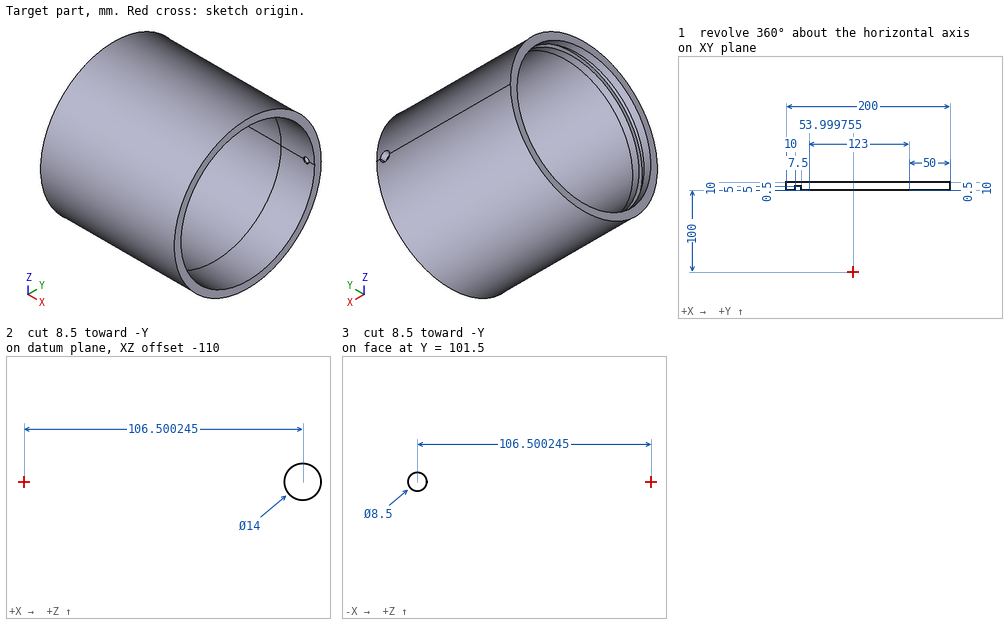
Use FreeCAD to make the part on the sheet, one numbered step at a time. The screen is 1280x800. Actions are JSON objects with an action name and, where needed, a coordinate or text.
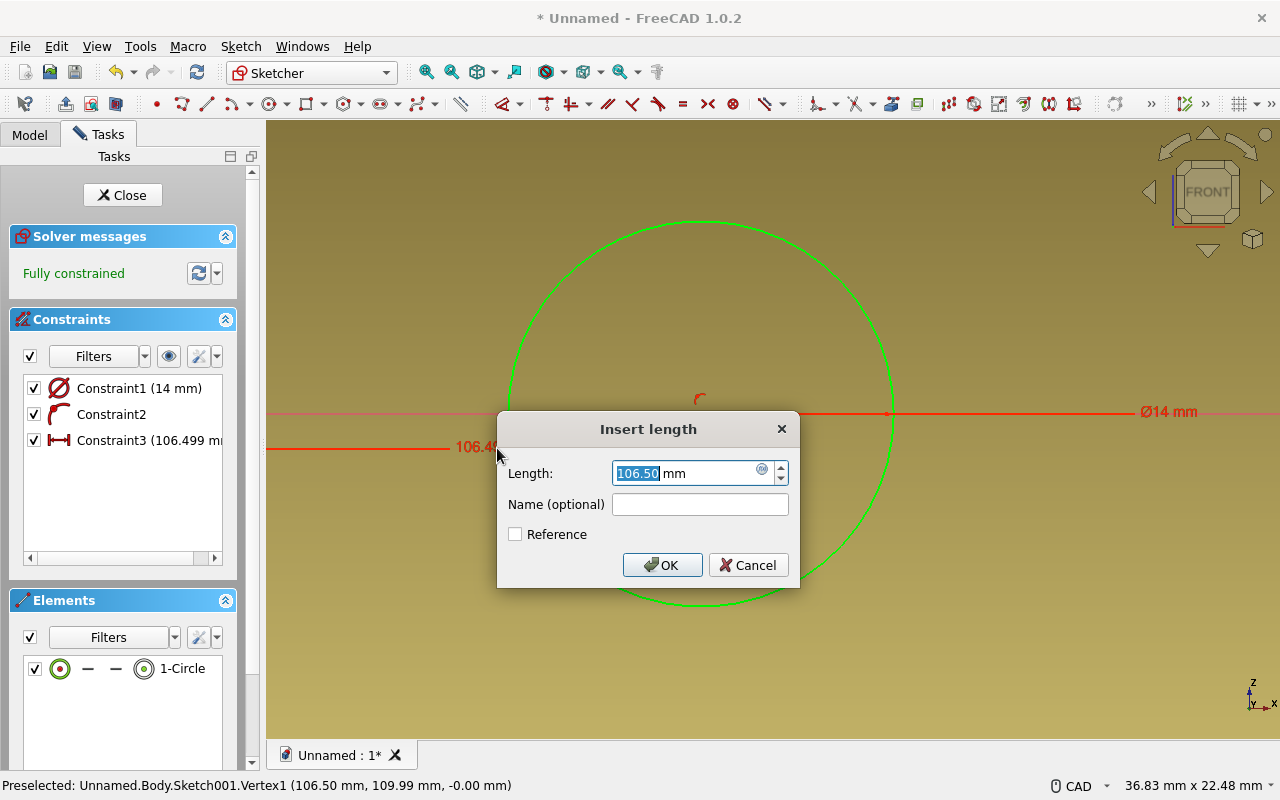
{"action": "type", "text": "106.500245"}
{"action": "key", "text": "Return"}
{"action": "key", "text": "Escape"}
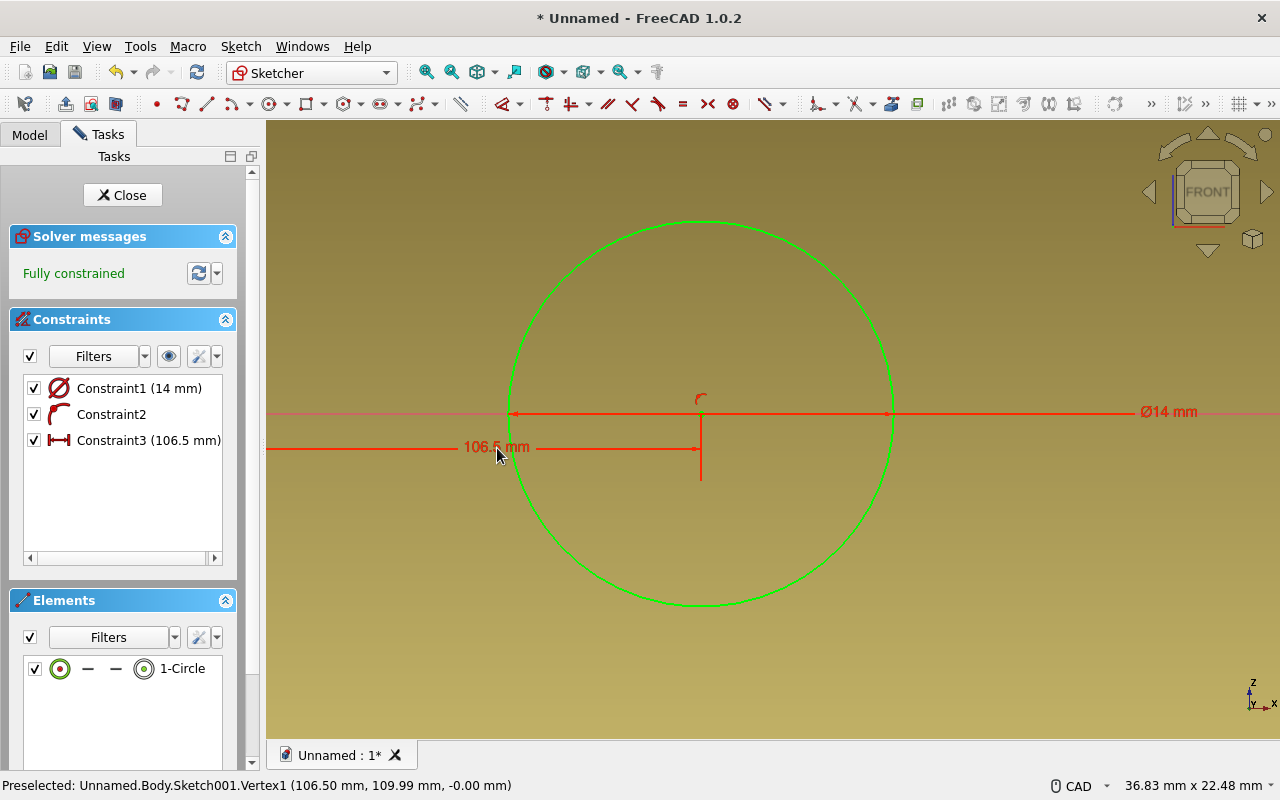
{"action": "left_click", "coordinate": [123, 195]}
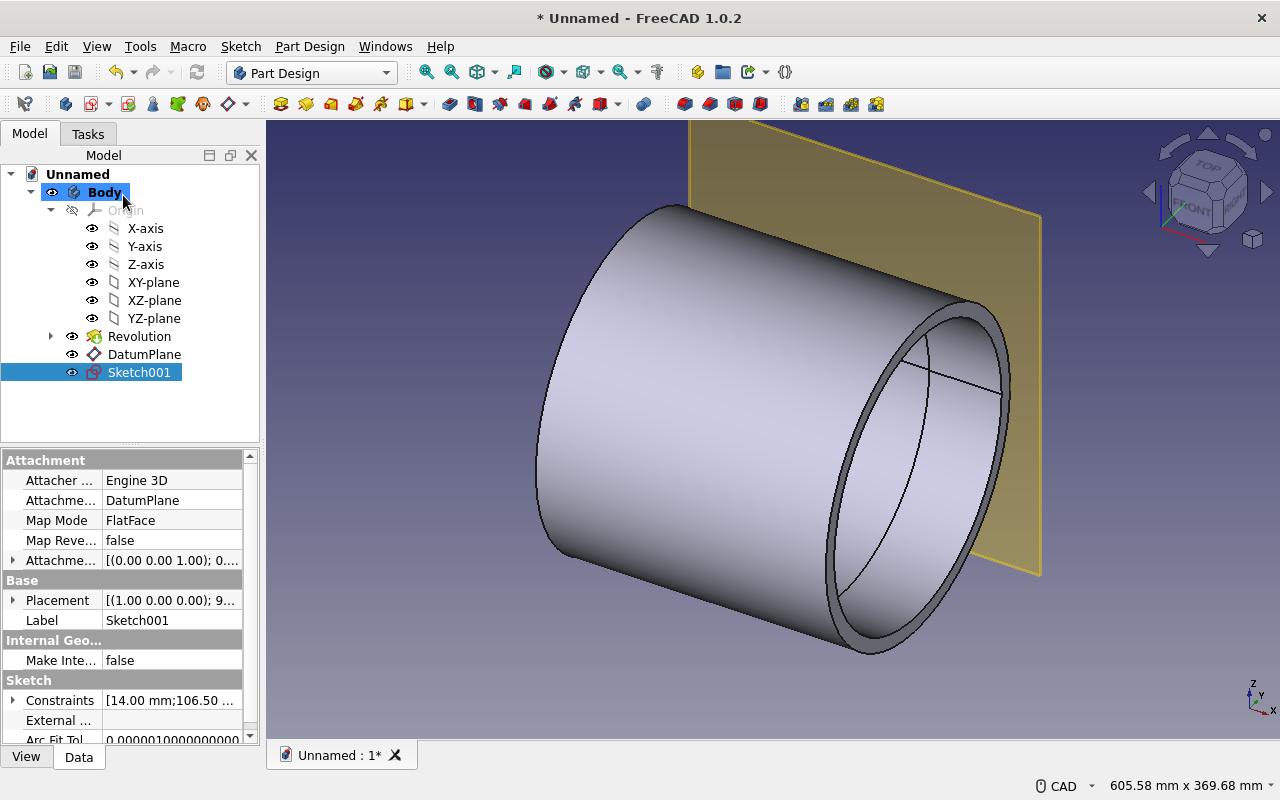
{"action": "left_click", "coordinate": [450, 104]}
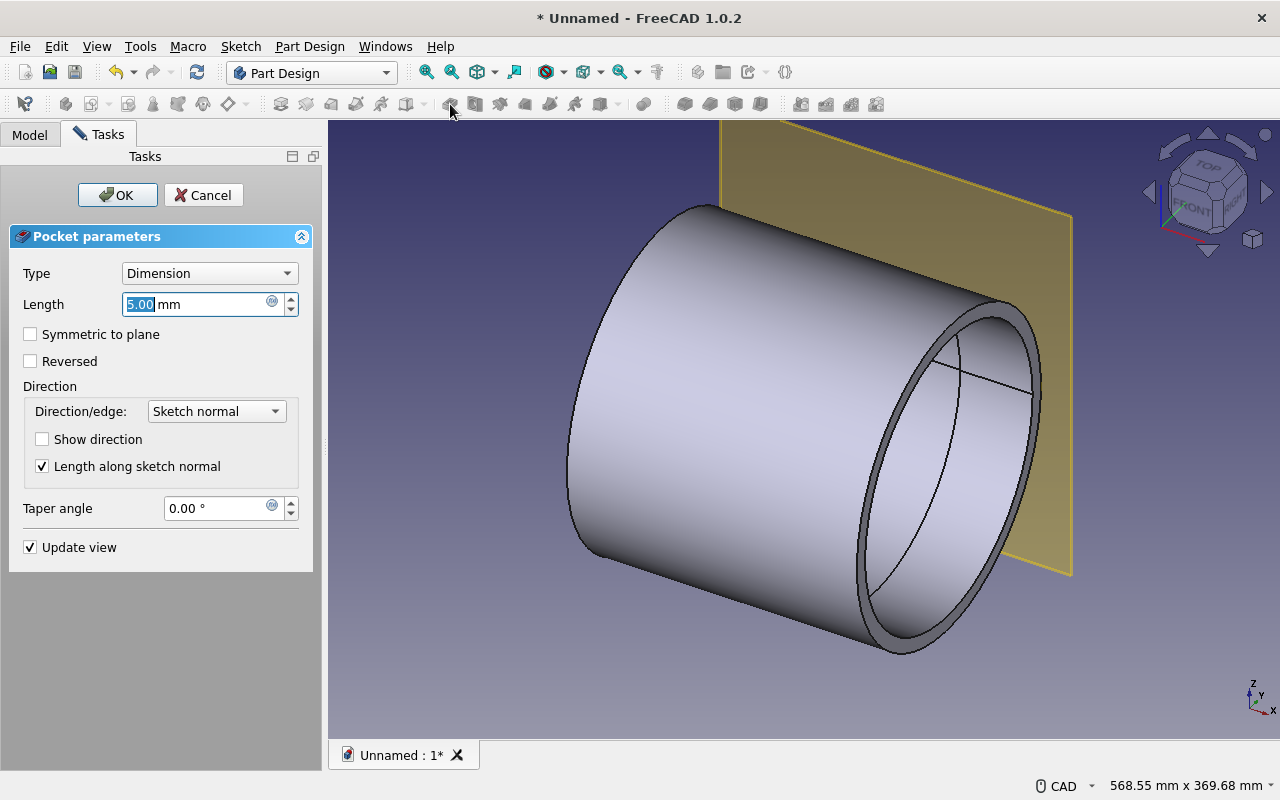
{"action": "type", "text": "8.5"}
{"action": "key", "text": "Tab"}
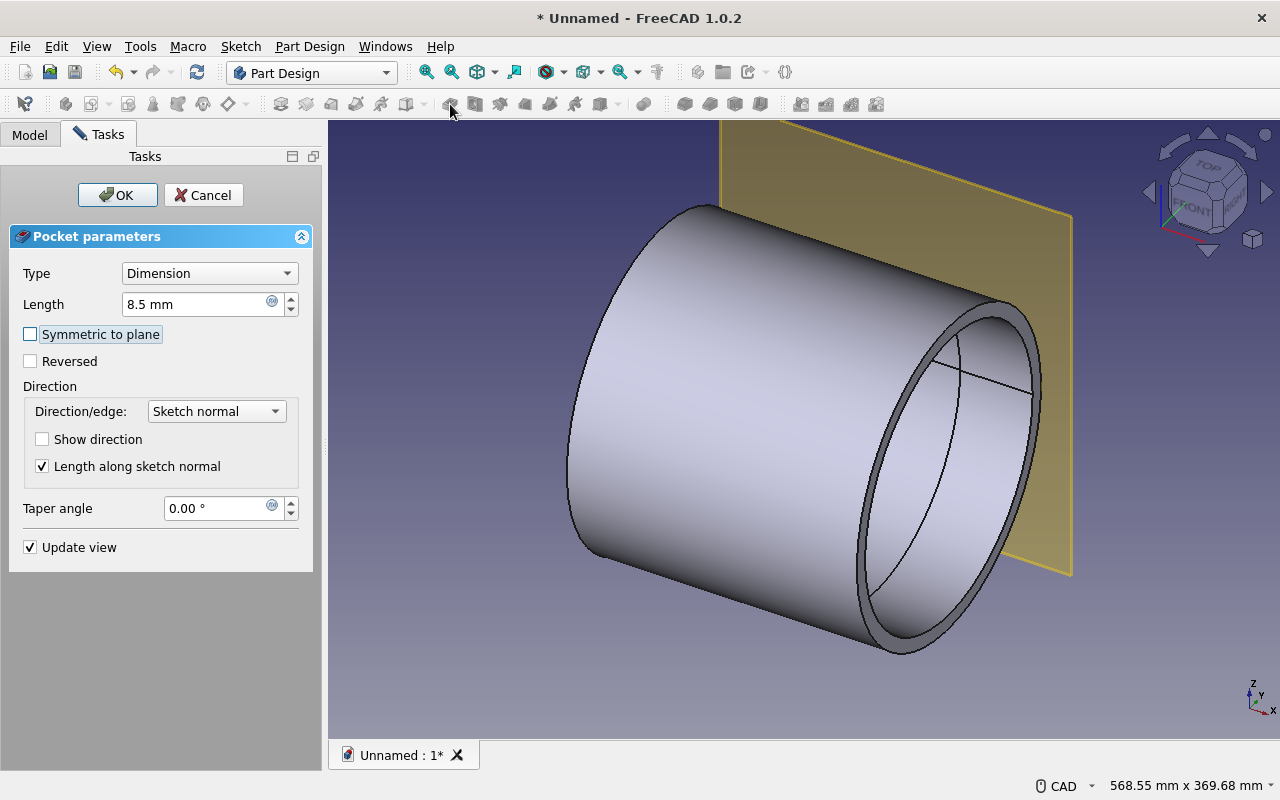
{"action": "left_click", "coordinate": [31, 361]}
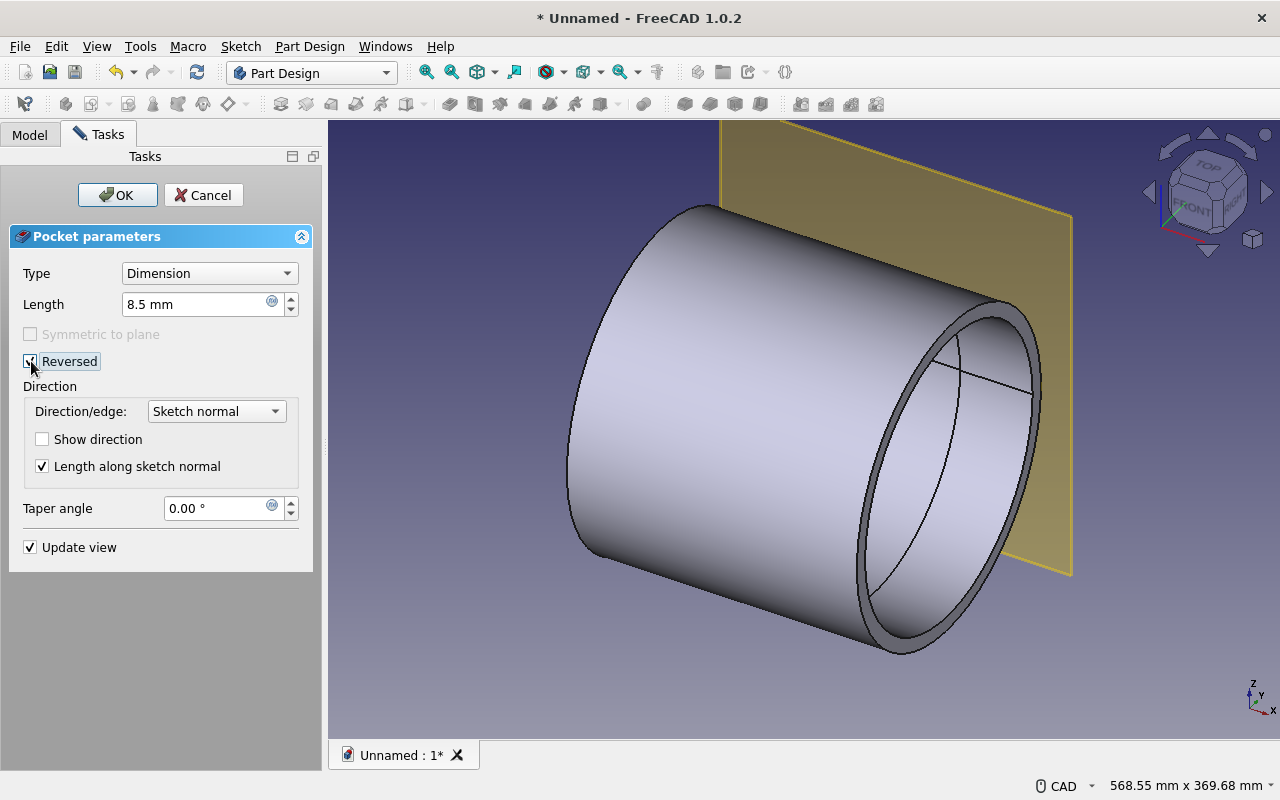
{"action": "left_click", "coordinate": [118, 195]}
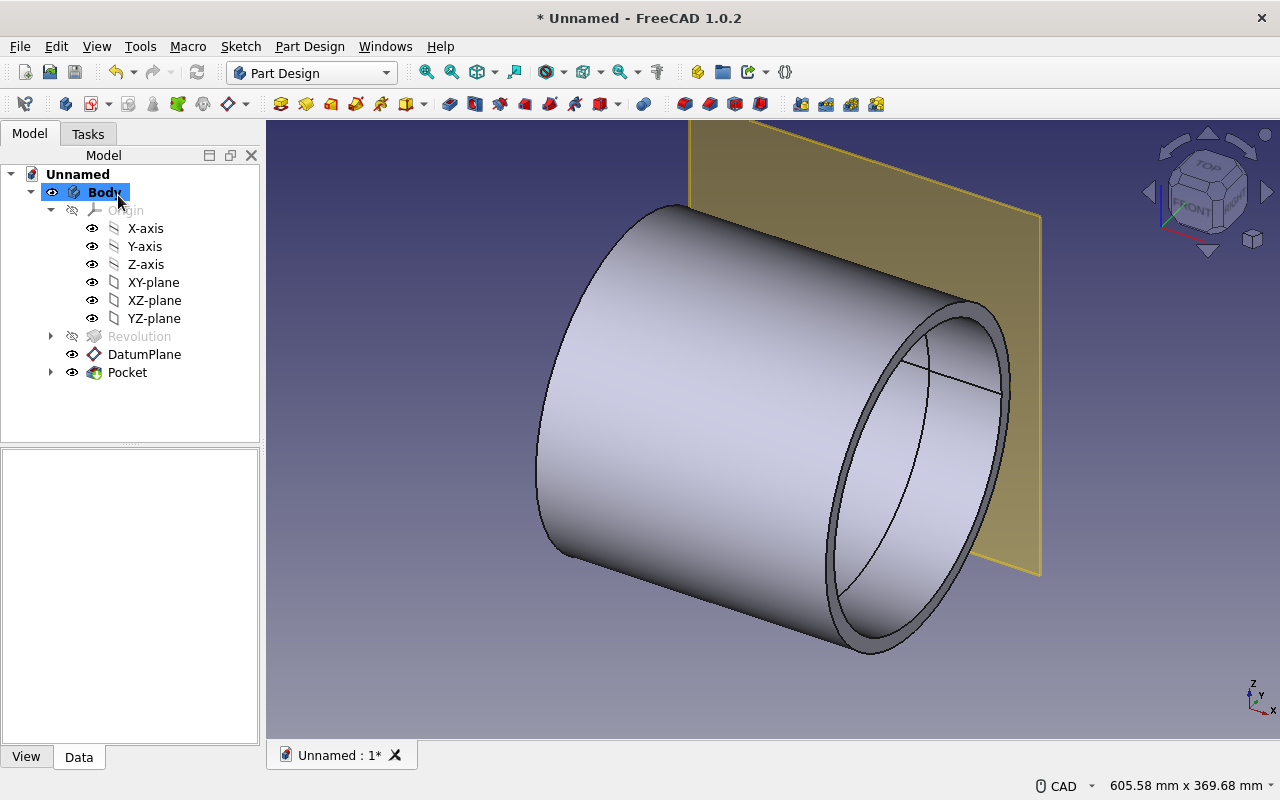
{"action": "left_click", "coordinate": [117, 354]}
{"action": "key", "text": "space"}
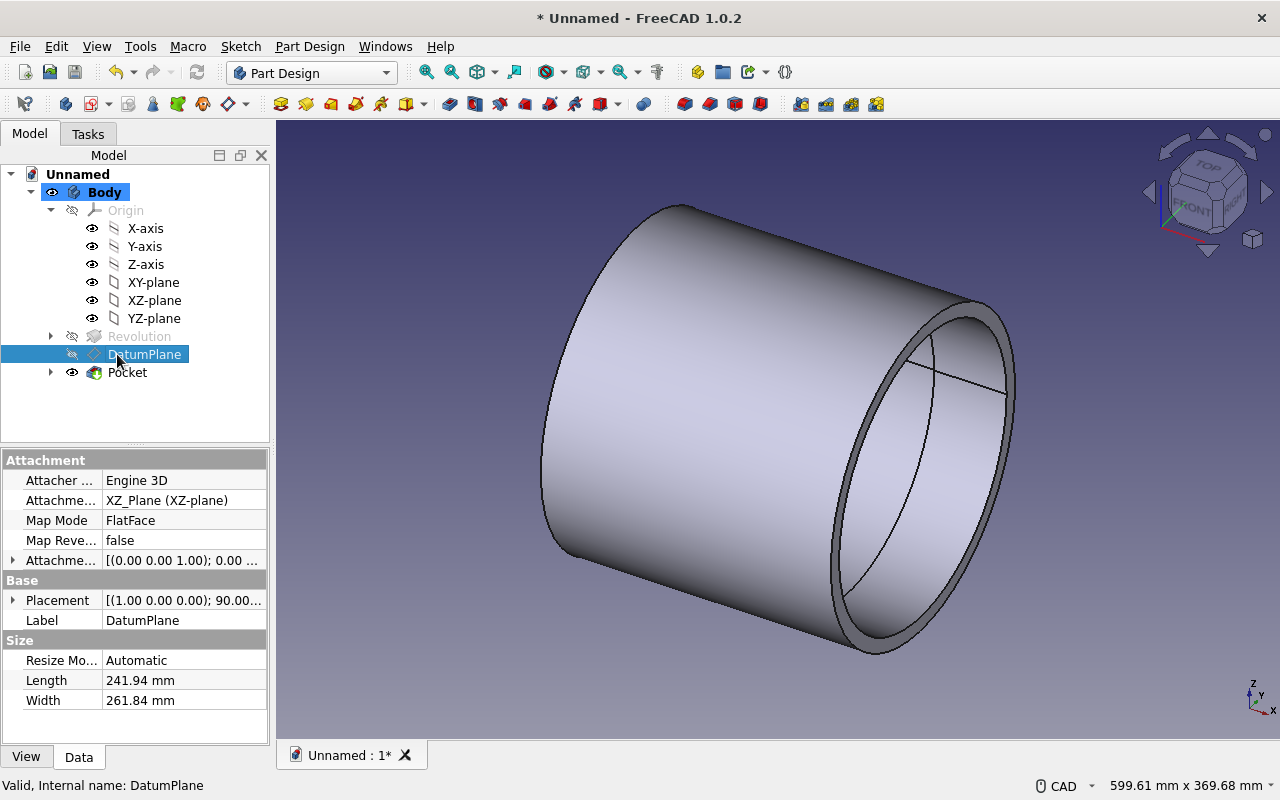
{"action": "key", "text": "4"}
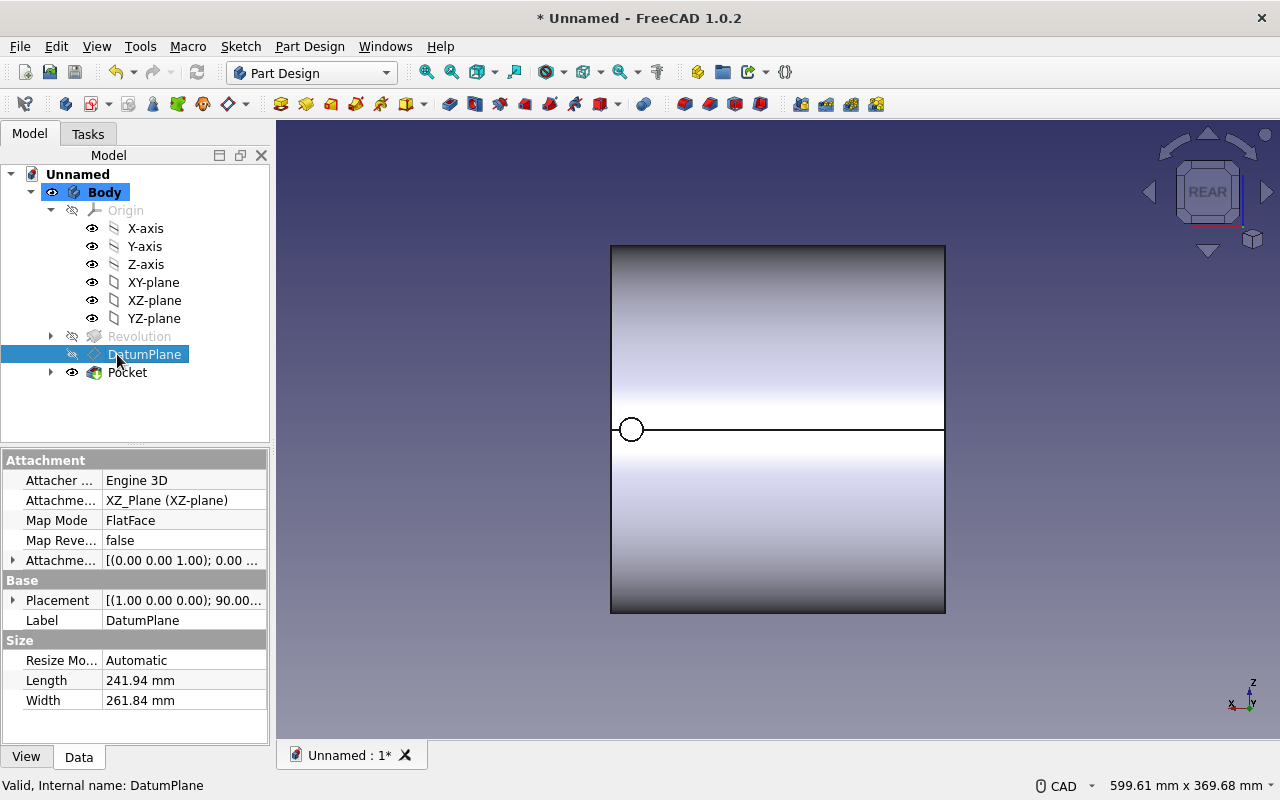
{"action": "left_click", "coordinate": [631, 429]}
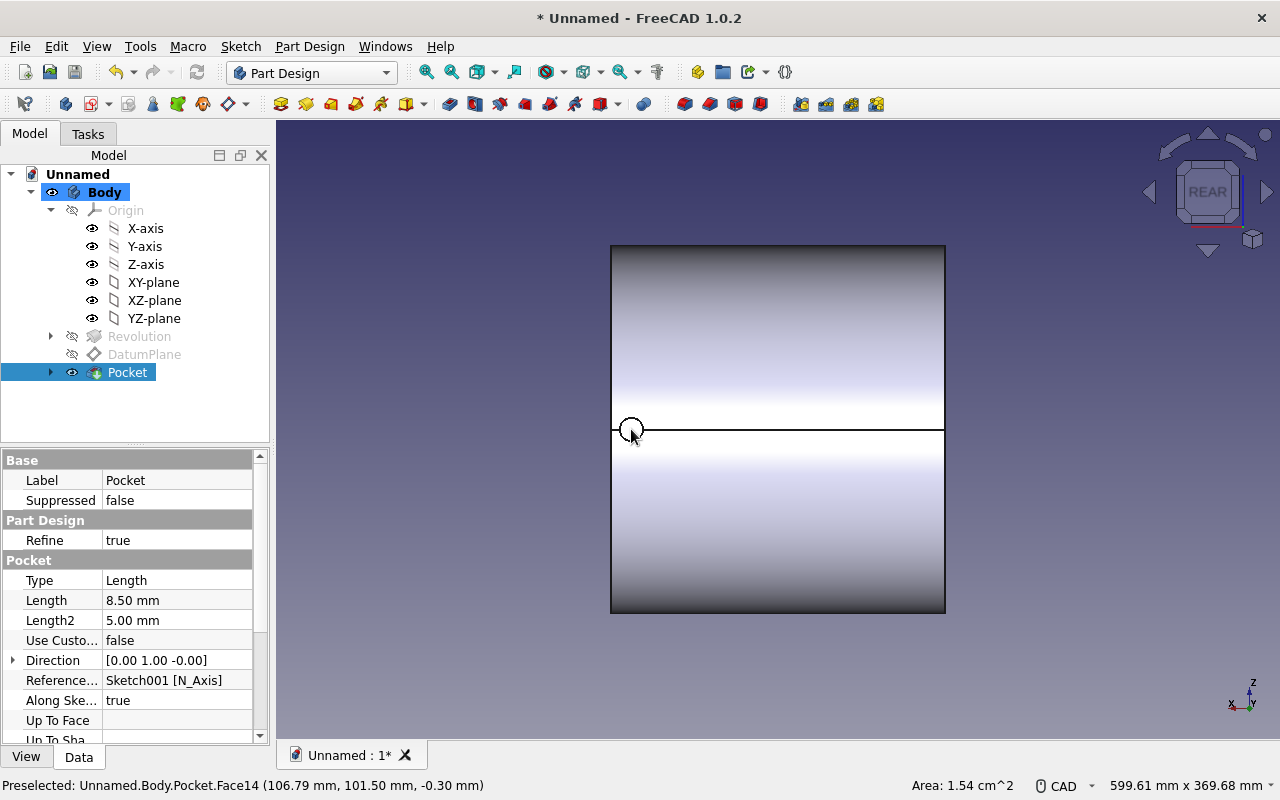
{"action": "left_click", "coordinate": [90, 104]}